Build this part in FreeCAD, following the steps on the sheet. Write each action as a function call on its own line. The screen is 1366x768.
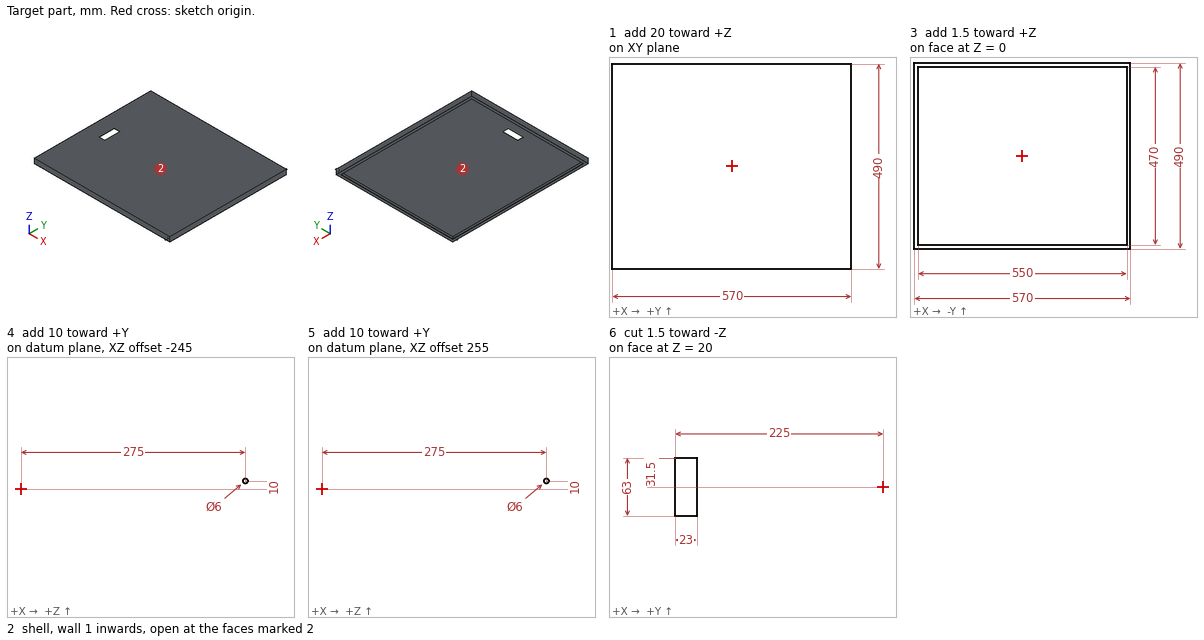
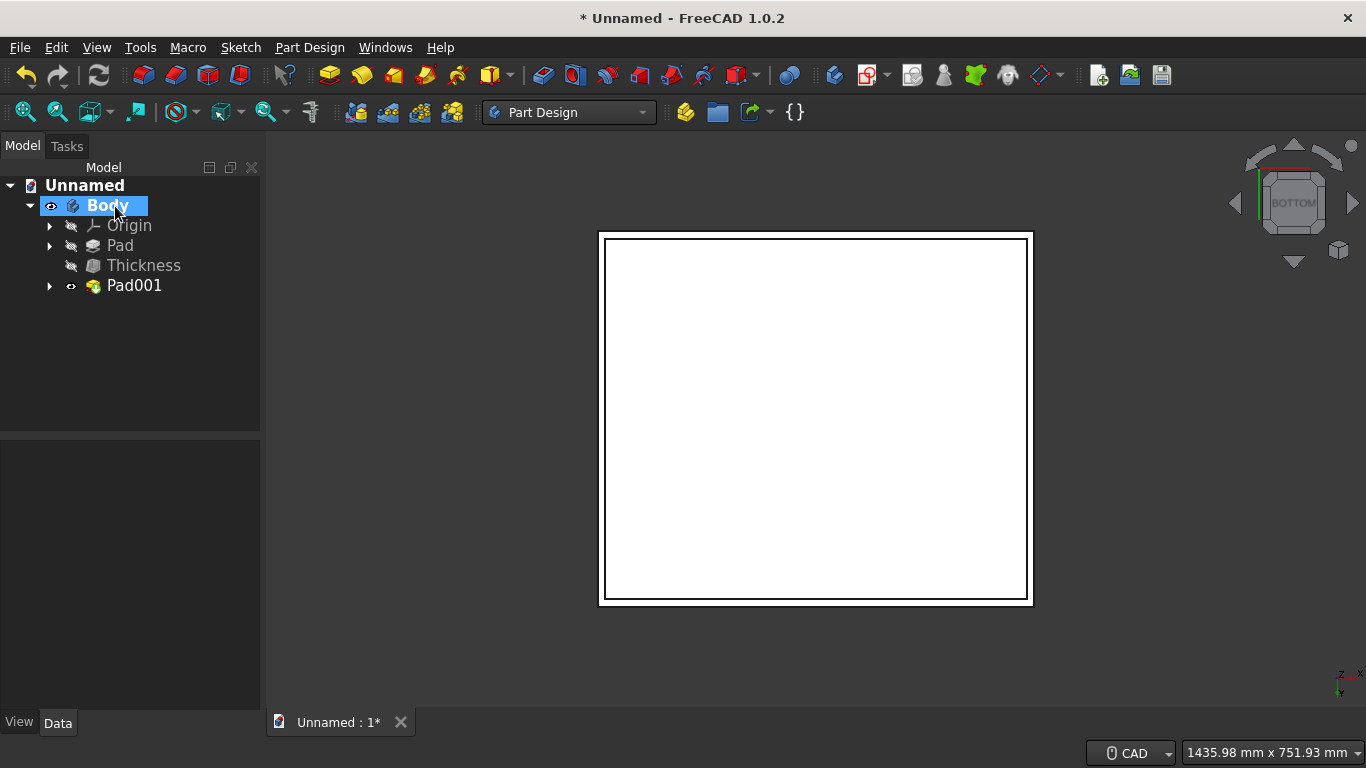
key(4)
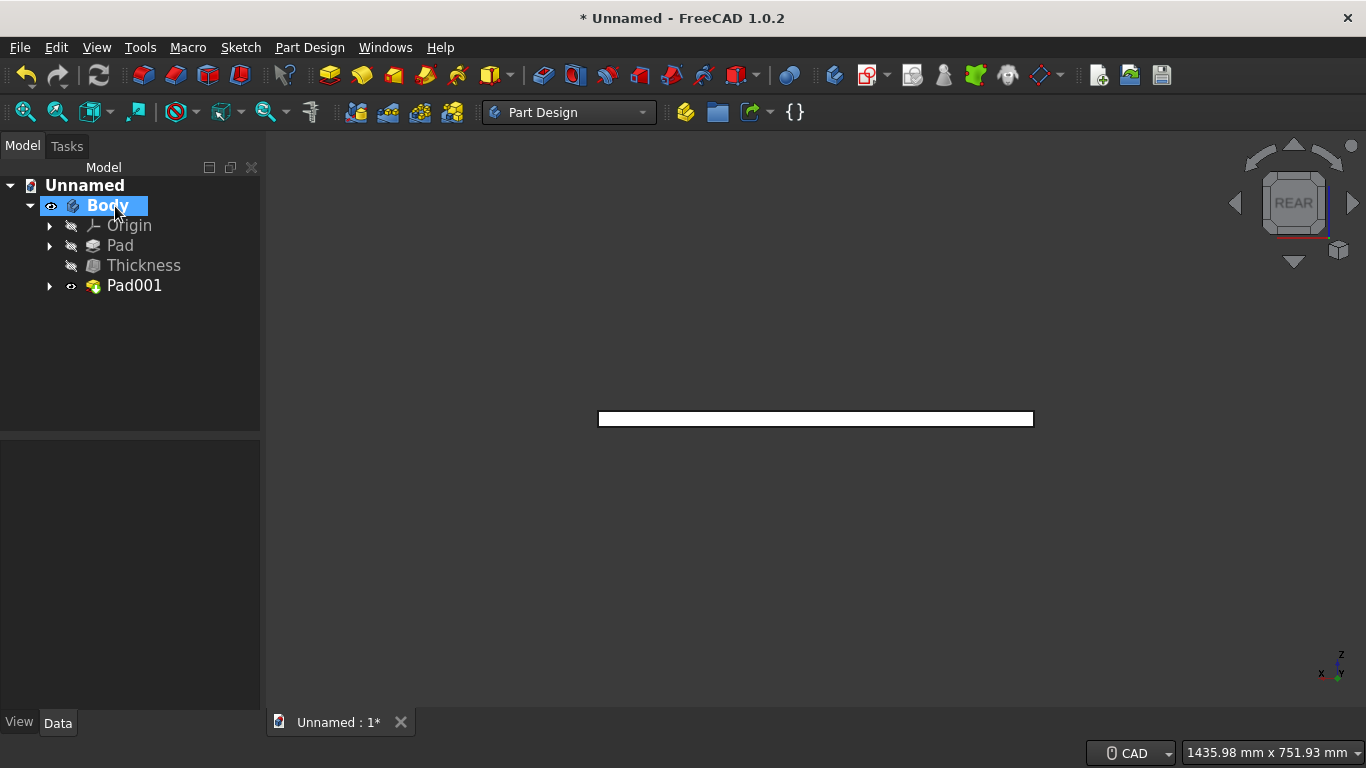
key(v)
key(f)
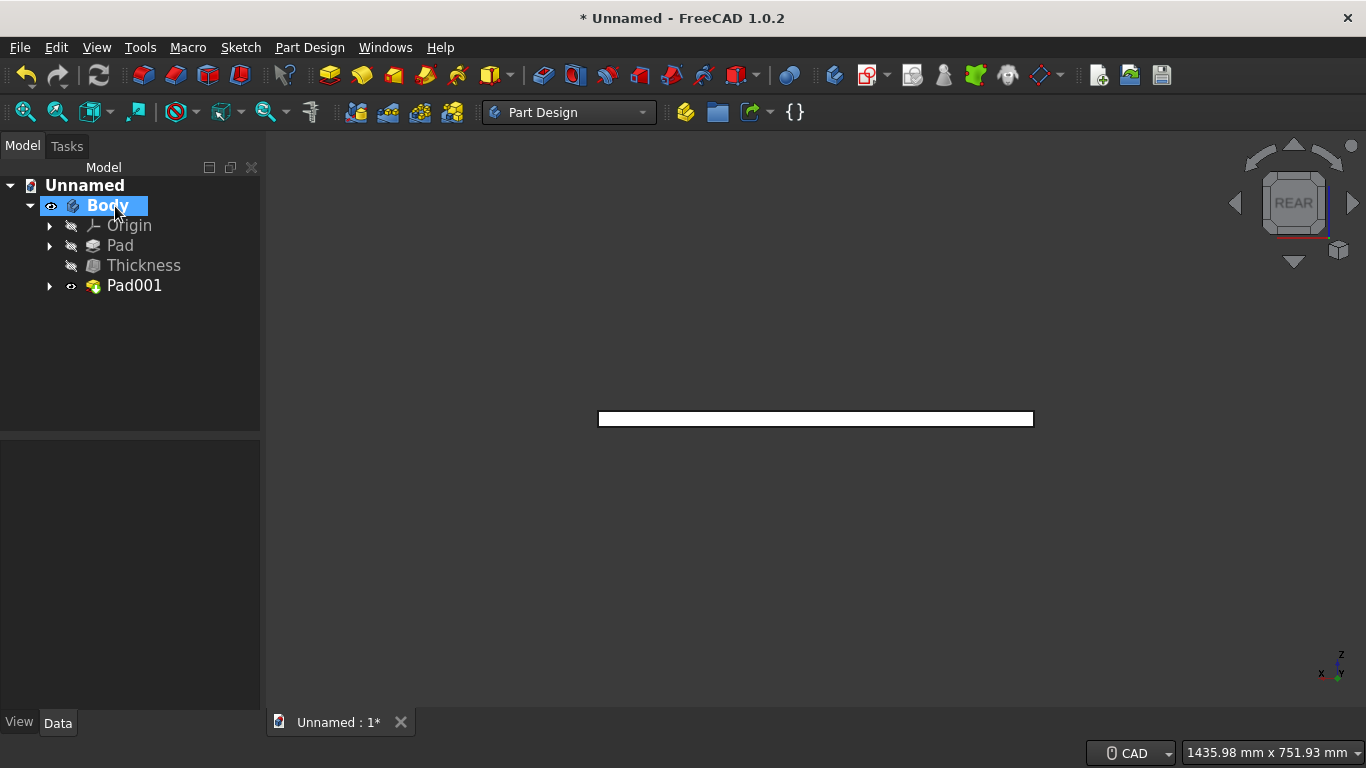
key(2)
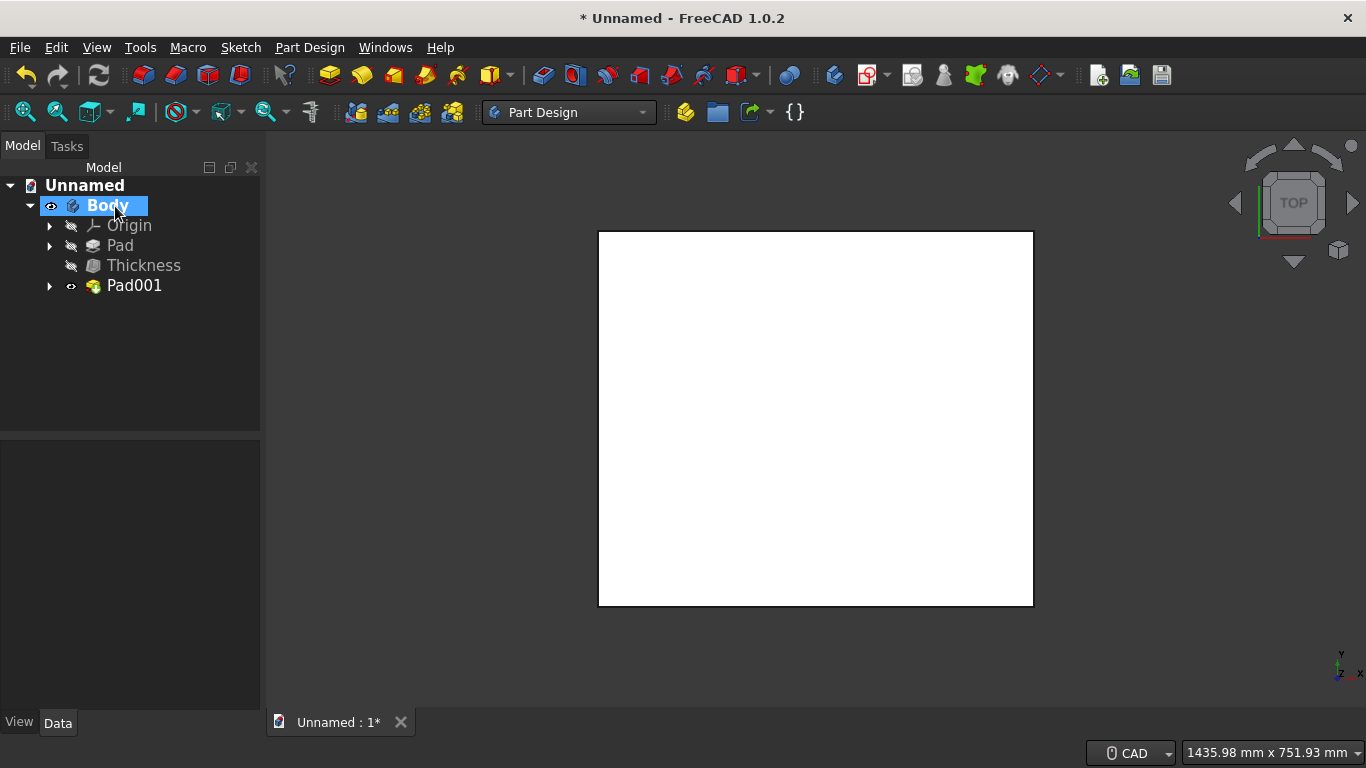
key(3)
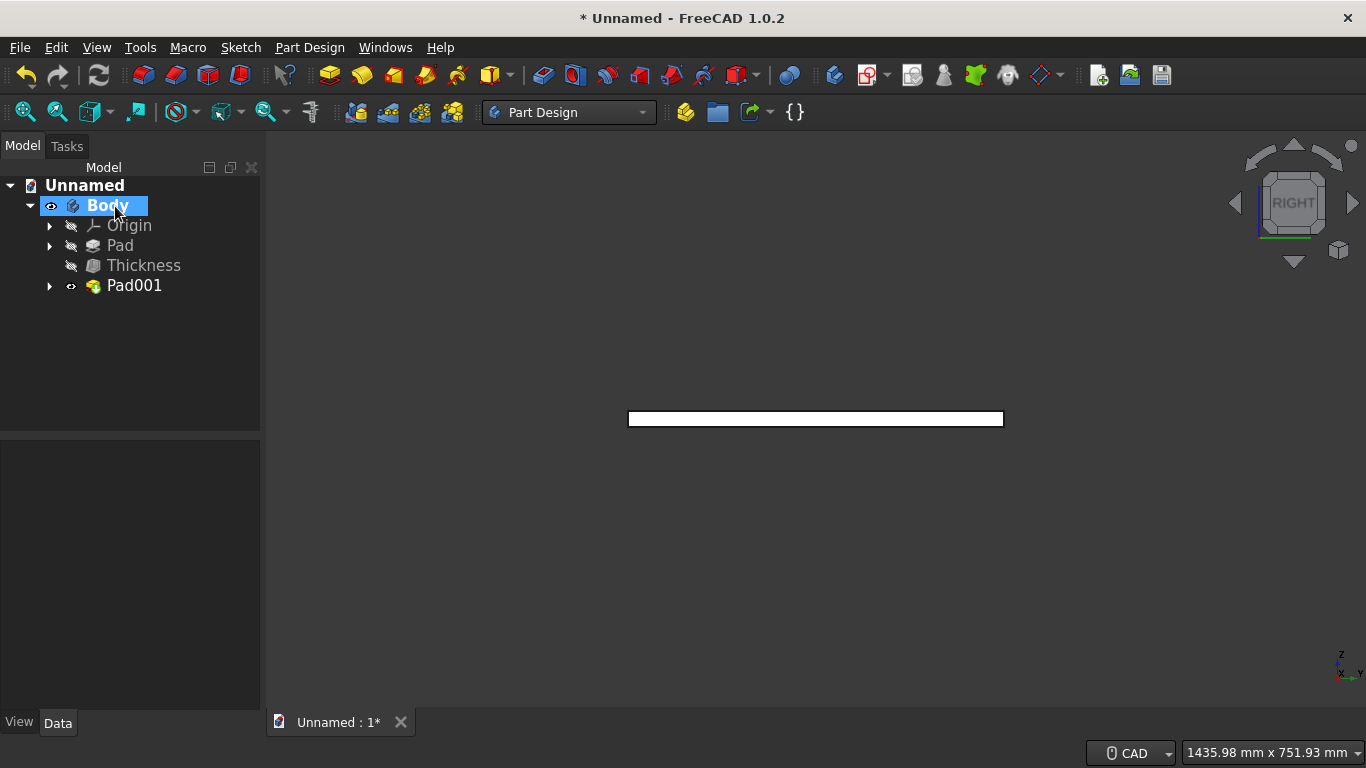
key(v)
key(f)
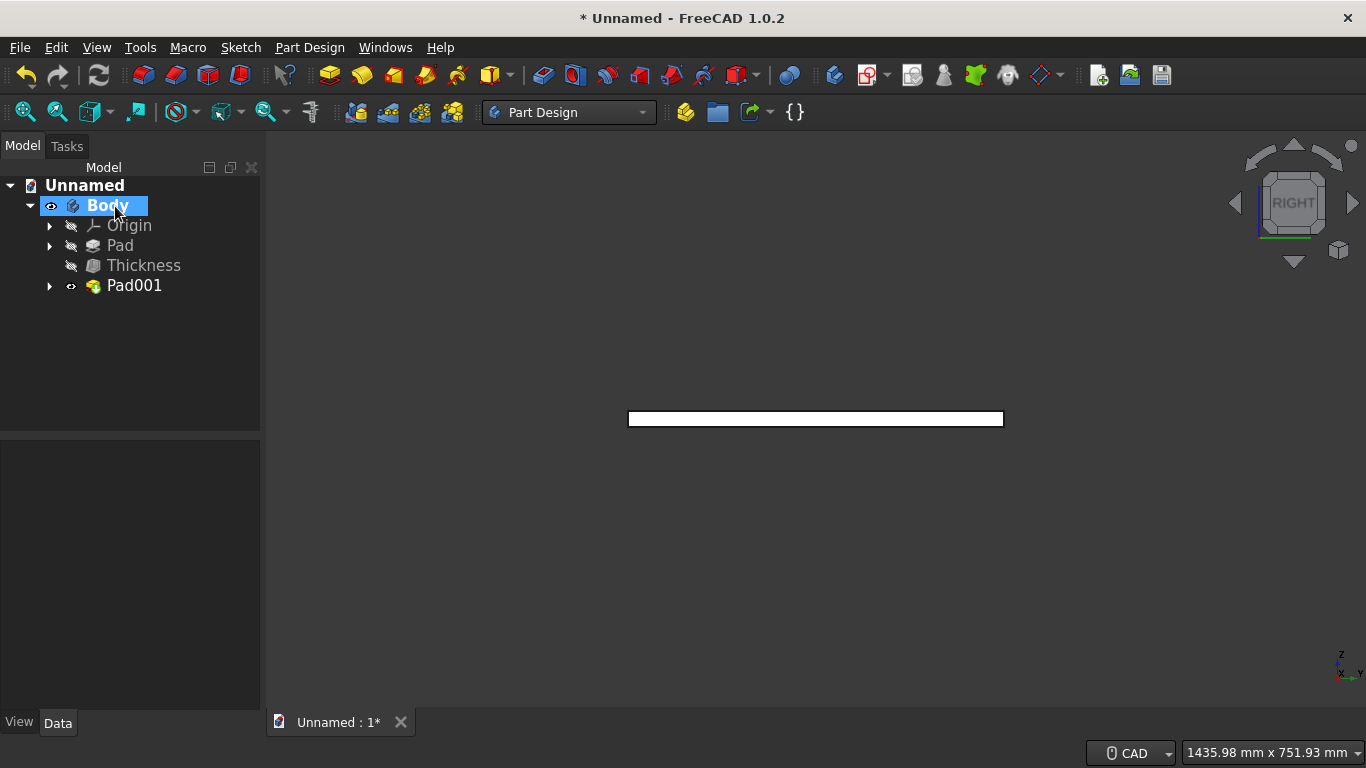
click(50, 226)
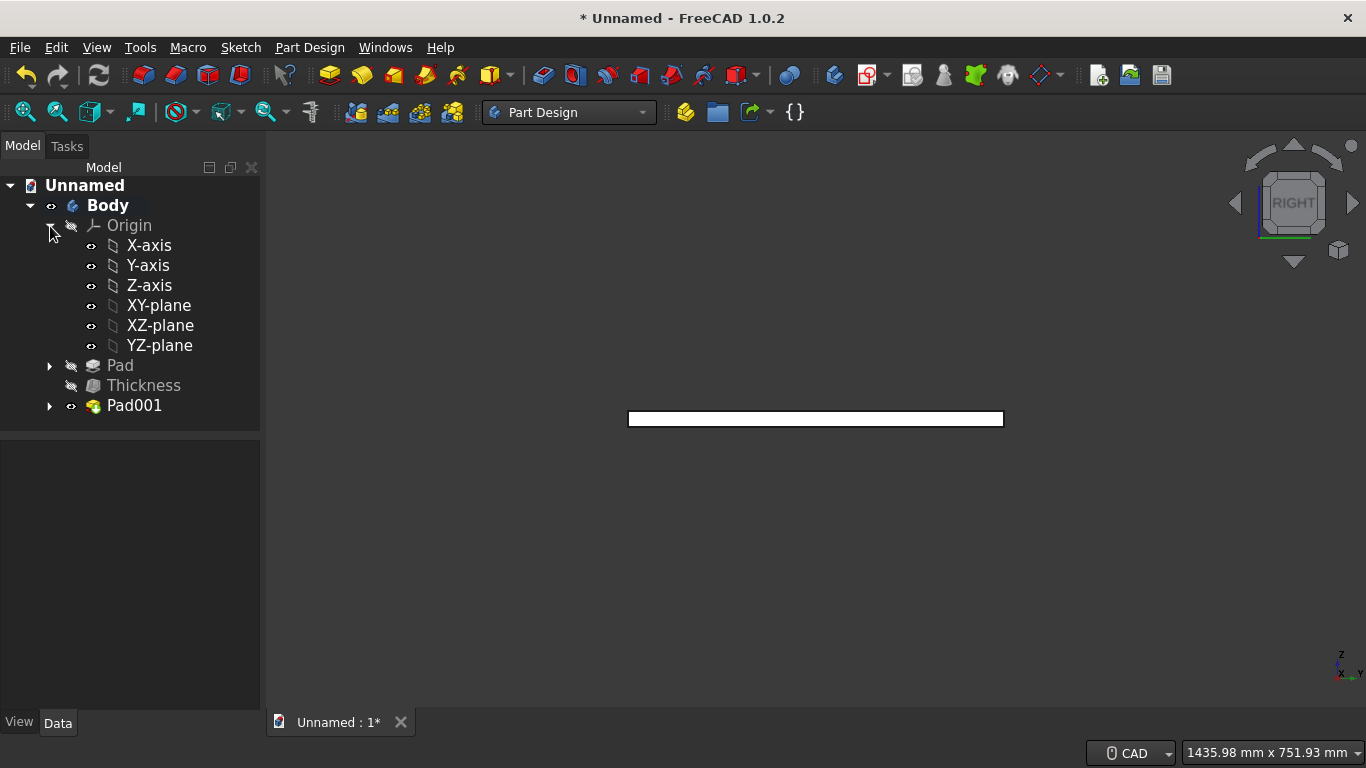
click(136, 326)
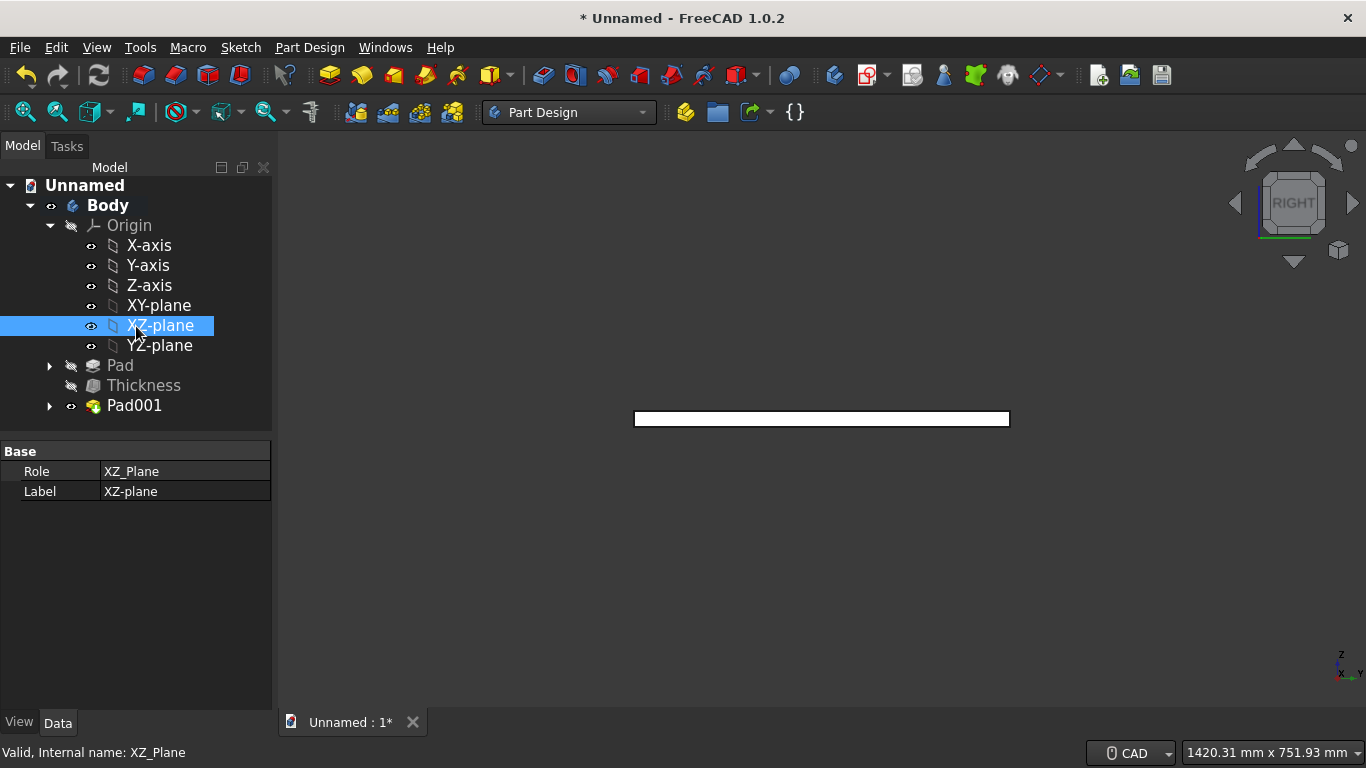
click(1040, 76)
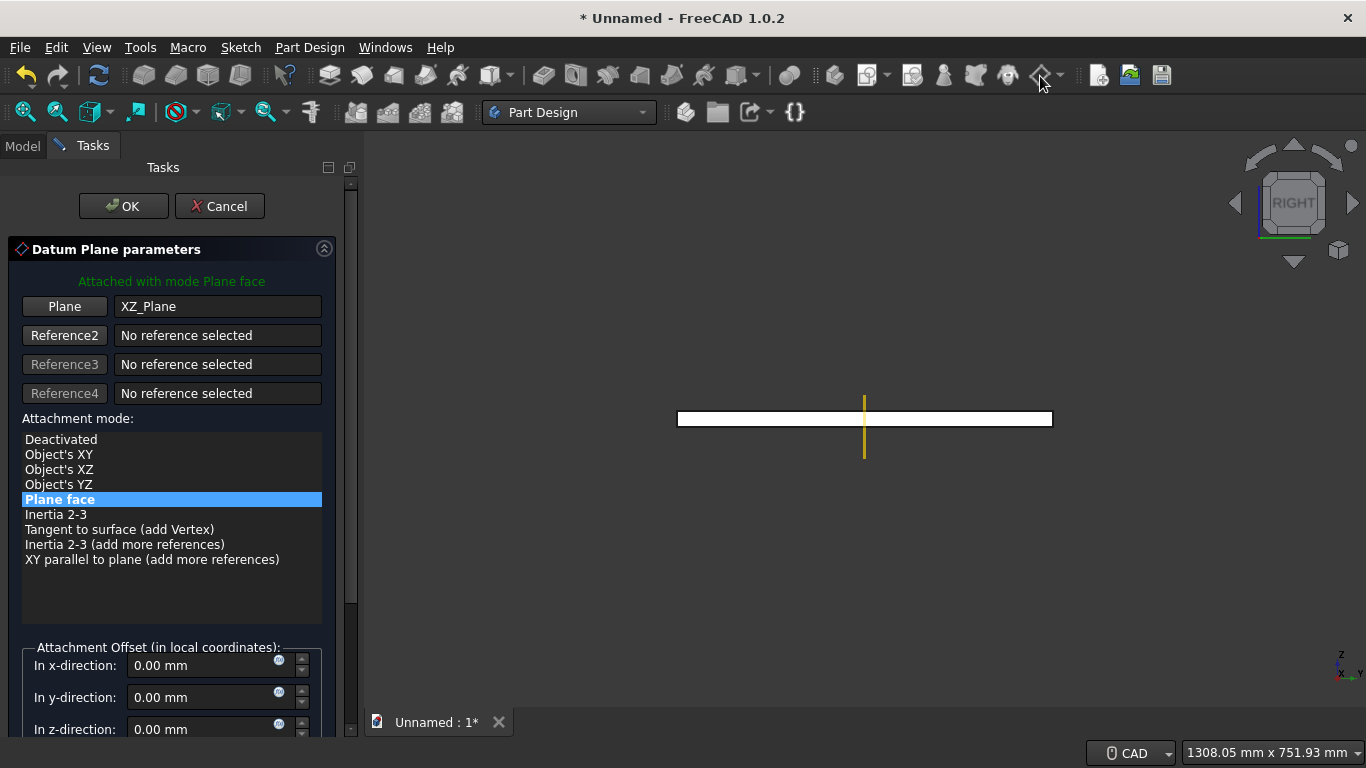
scroll(351, 456, down, 2)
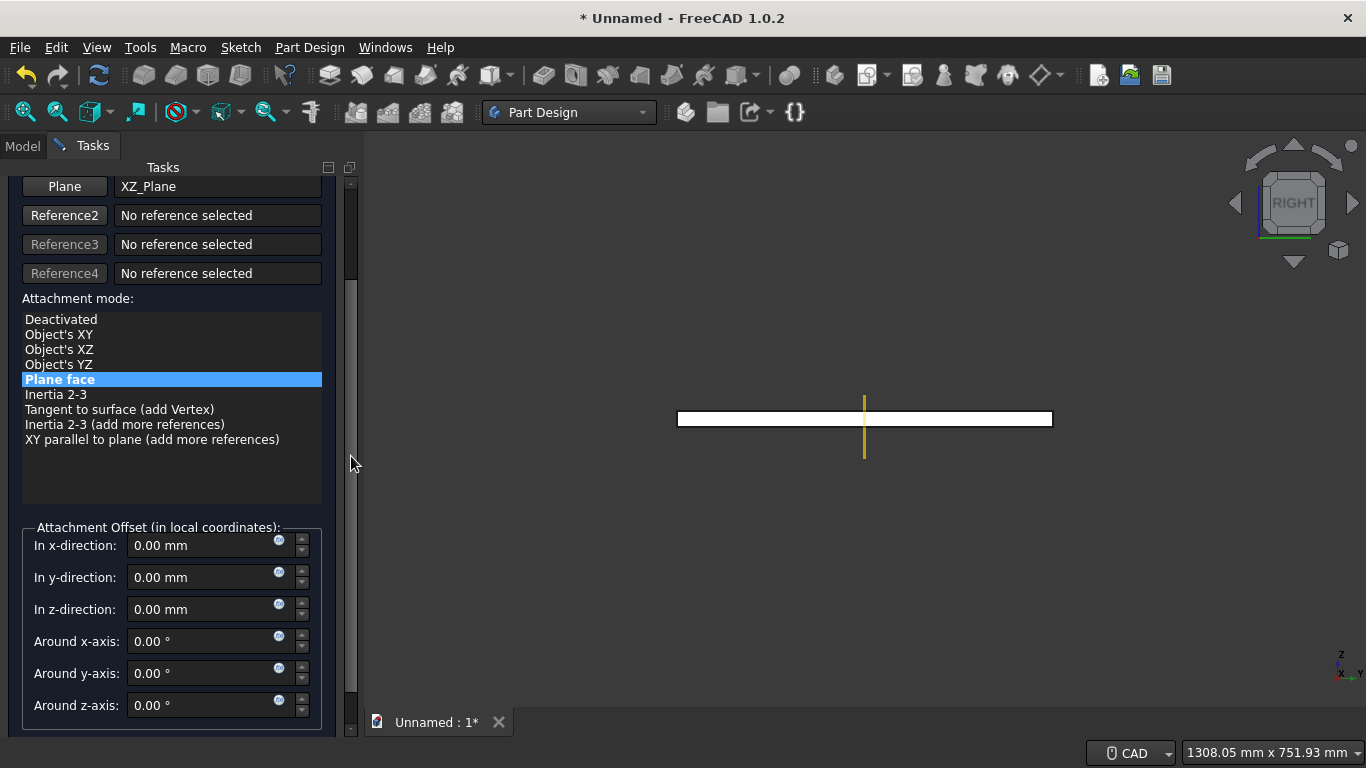
triple_click(210, 609)